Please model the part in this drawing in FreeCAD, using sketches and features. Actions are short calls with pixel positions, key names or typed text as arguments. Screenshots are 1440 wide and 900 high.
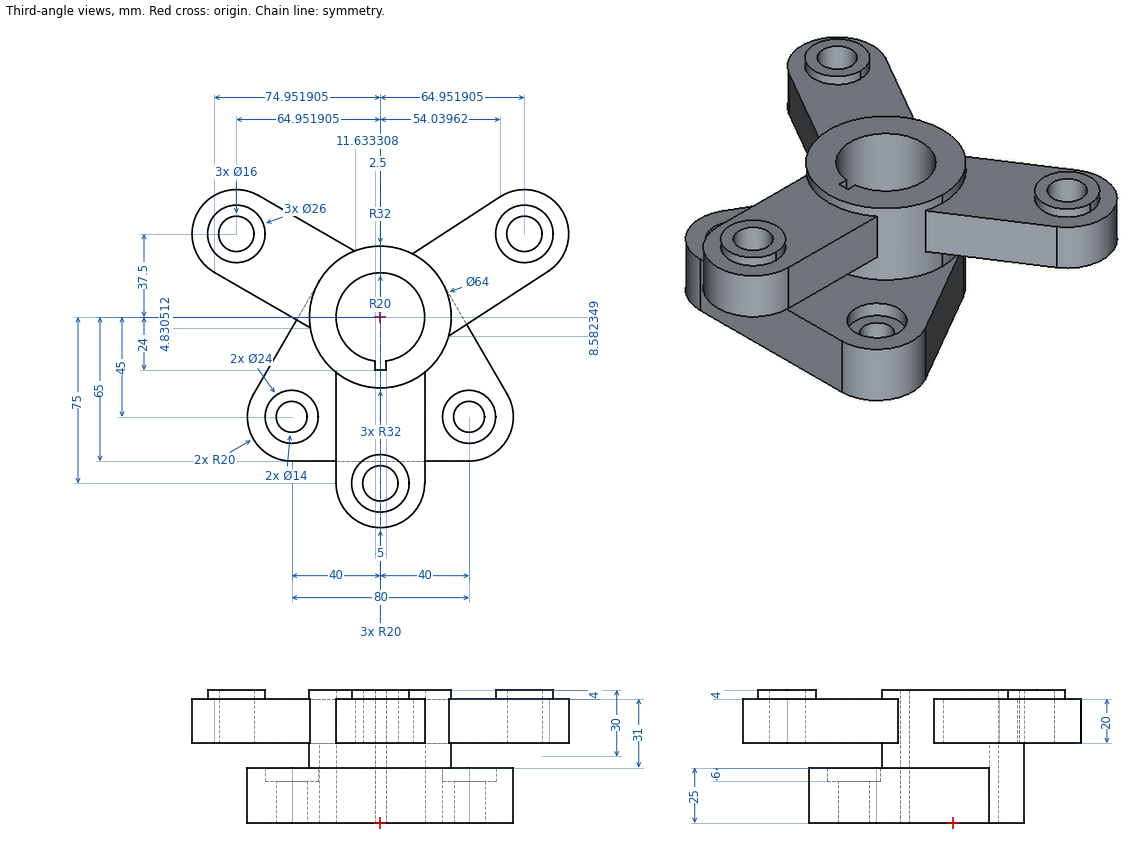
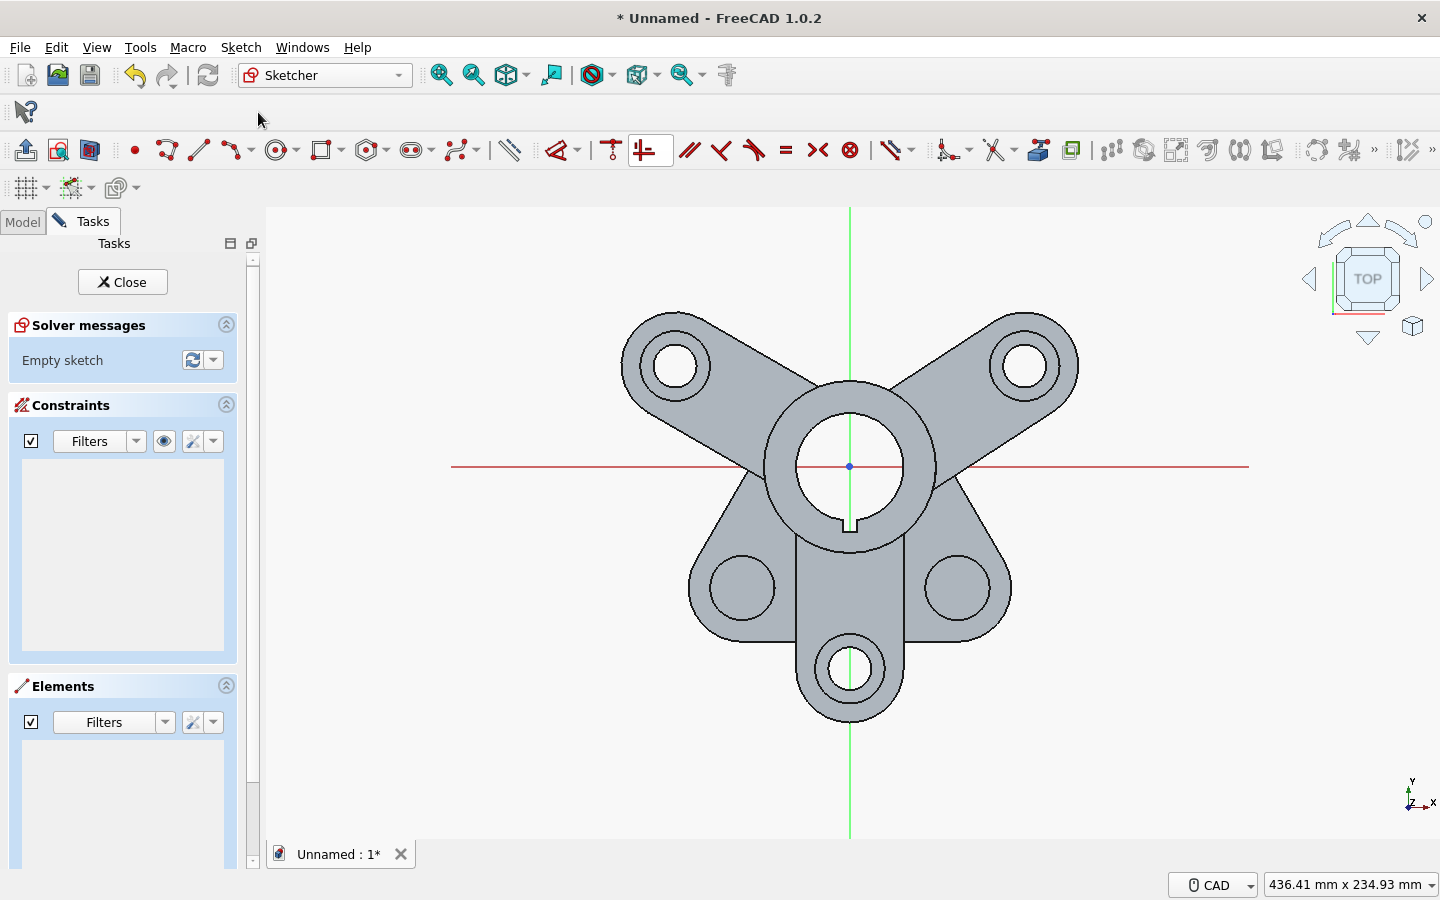
scroll(888, 545, up, 5)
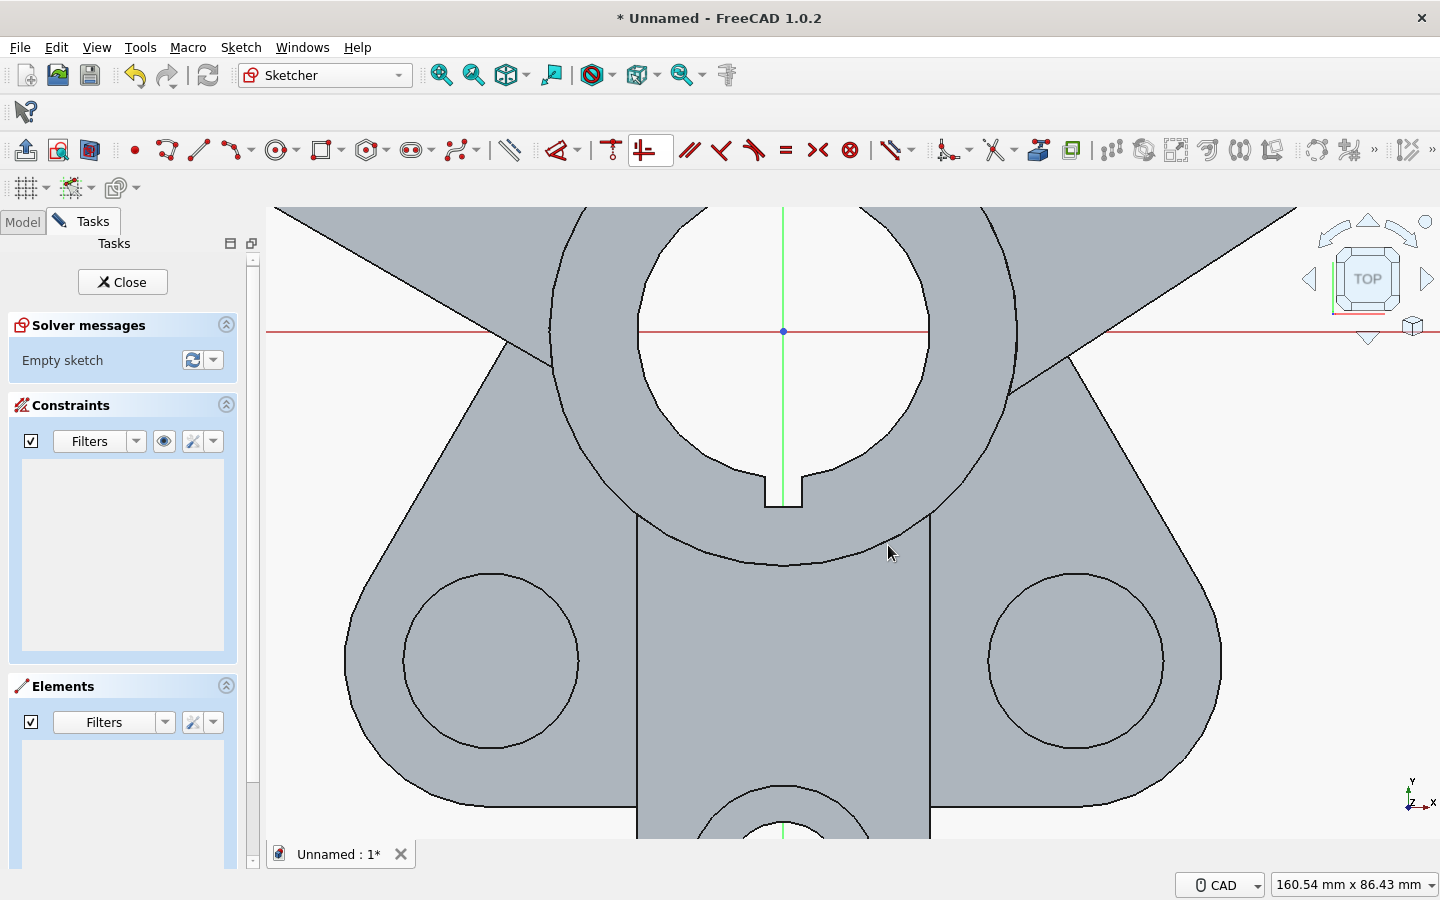
key(g)
key(c)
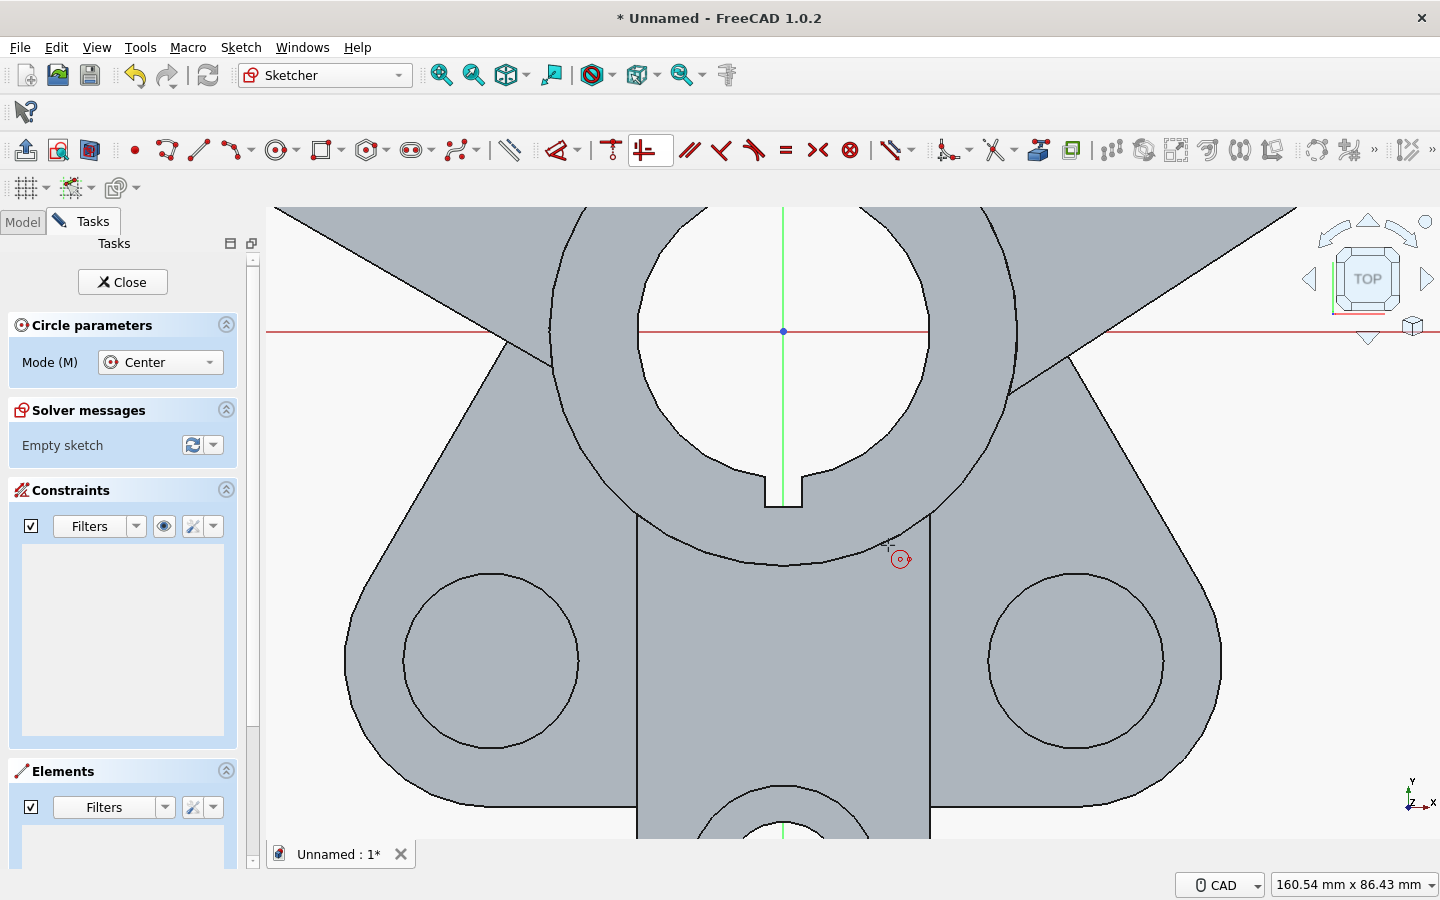
click(491, 661)
move(527, 625)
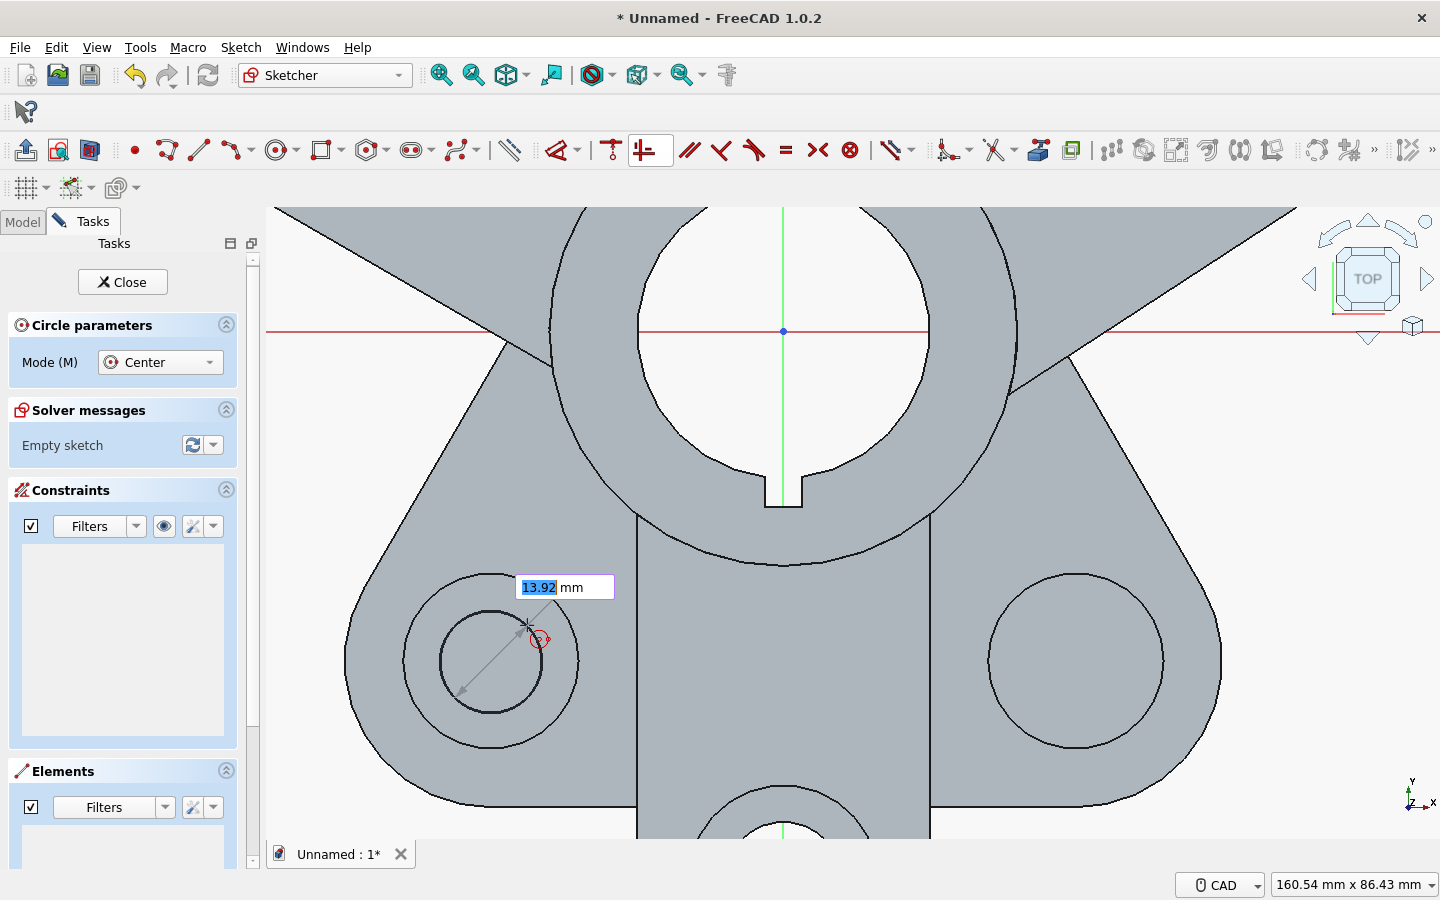
text(14)
key(Return)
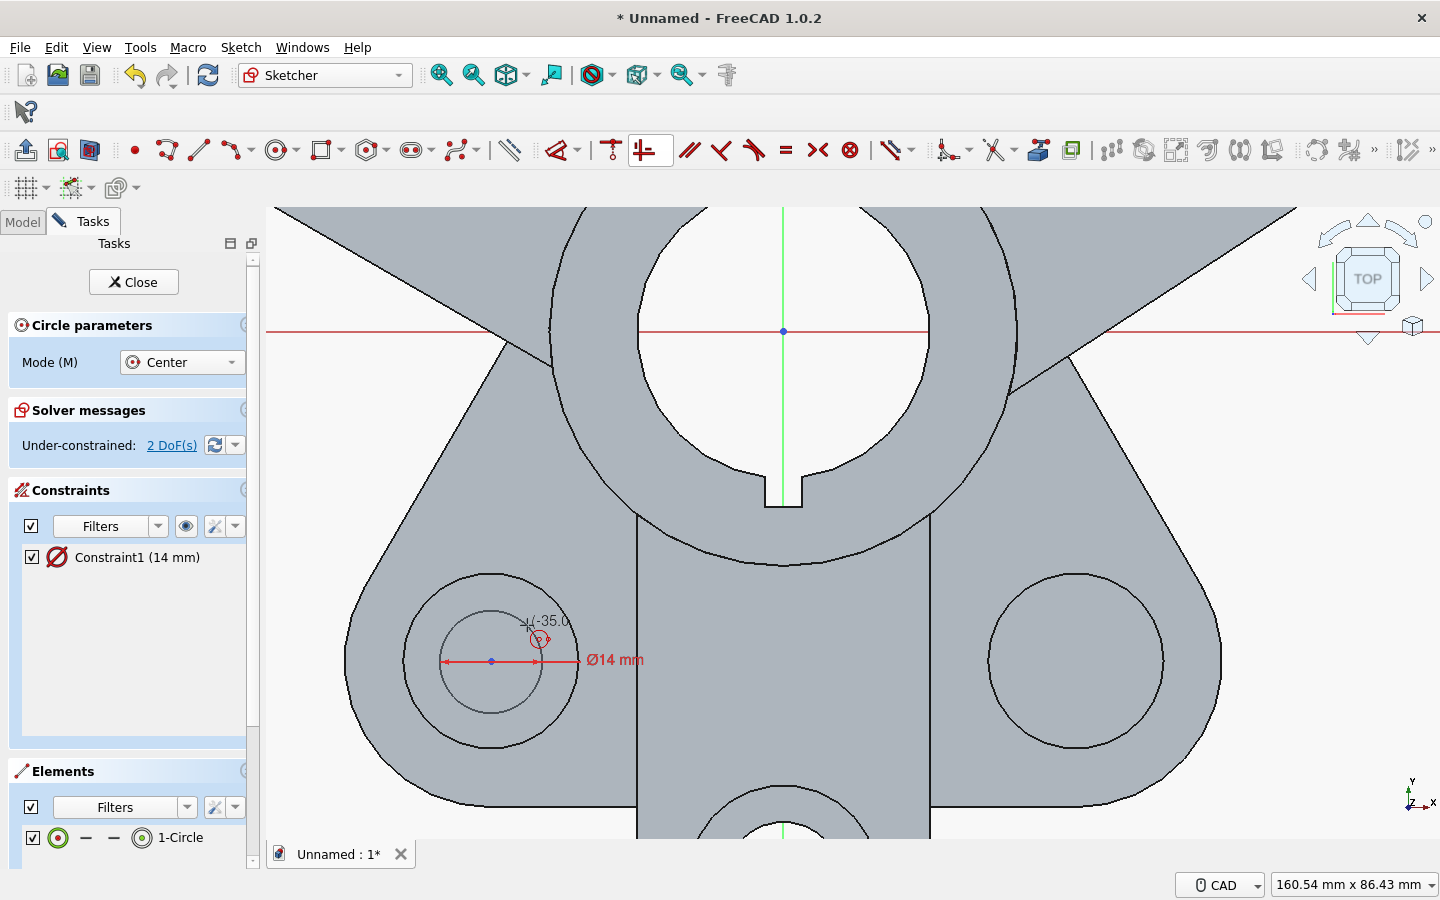
click(1076, 661)
move(1112, 625)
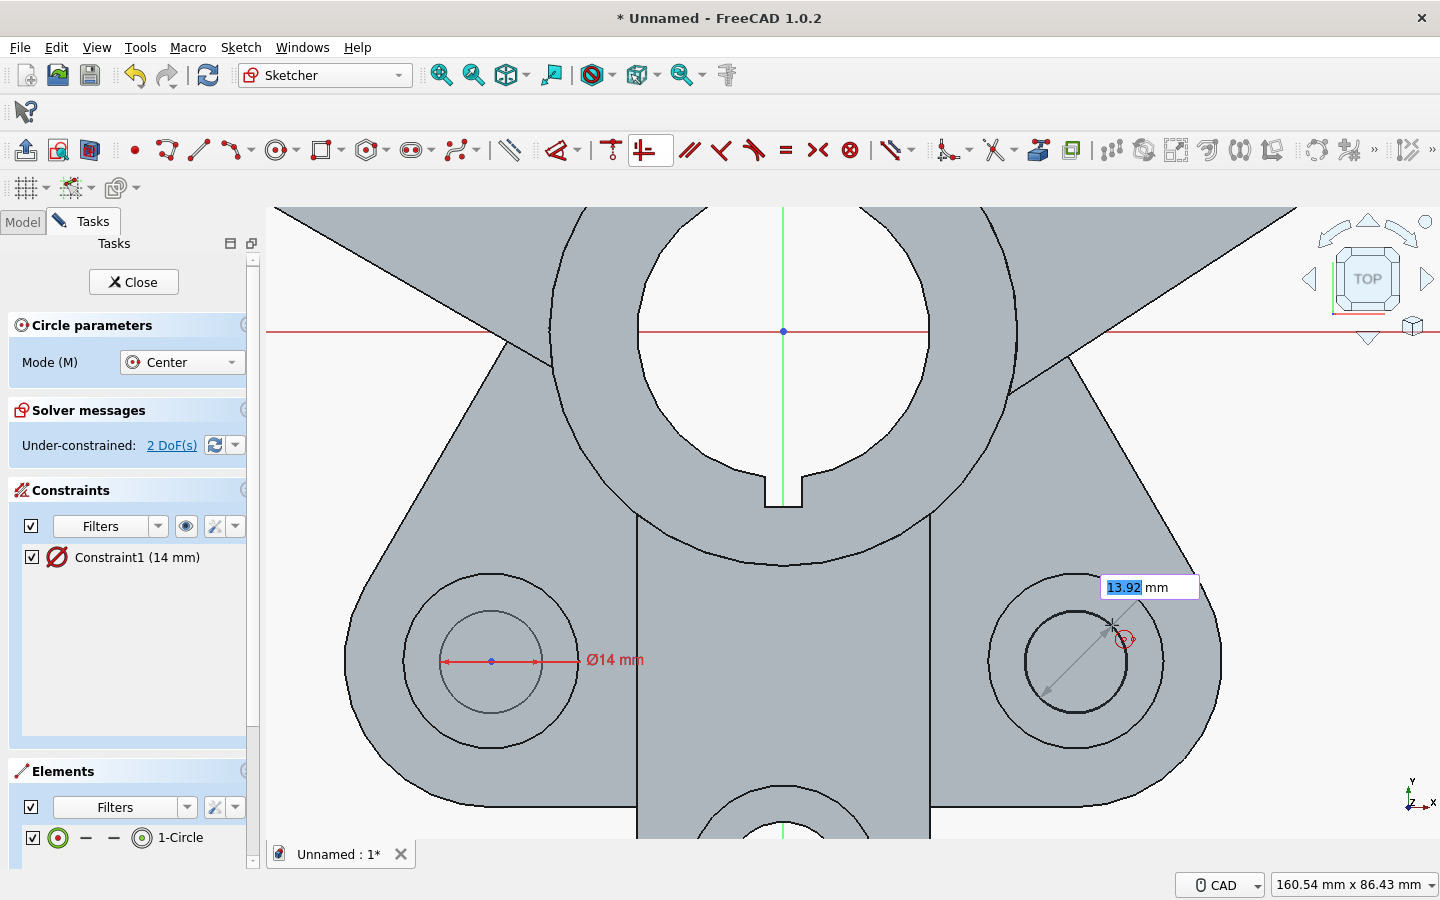
text(14)
key(Return)
key(Escape)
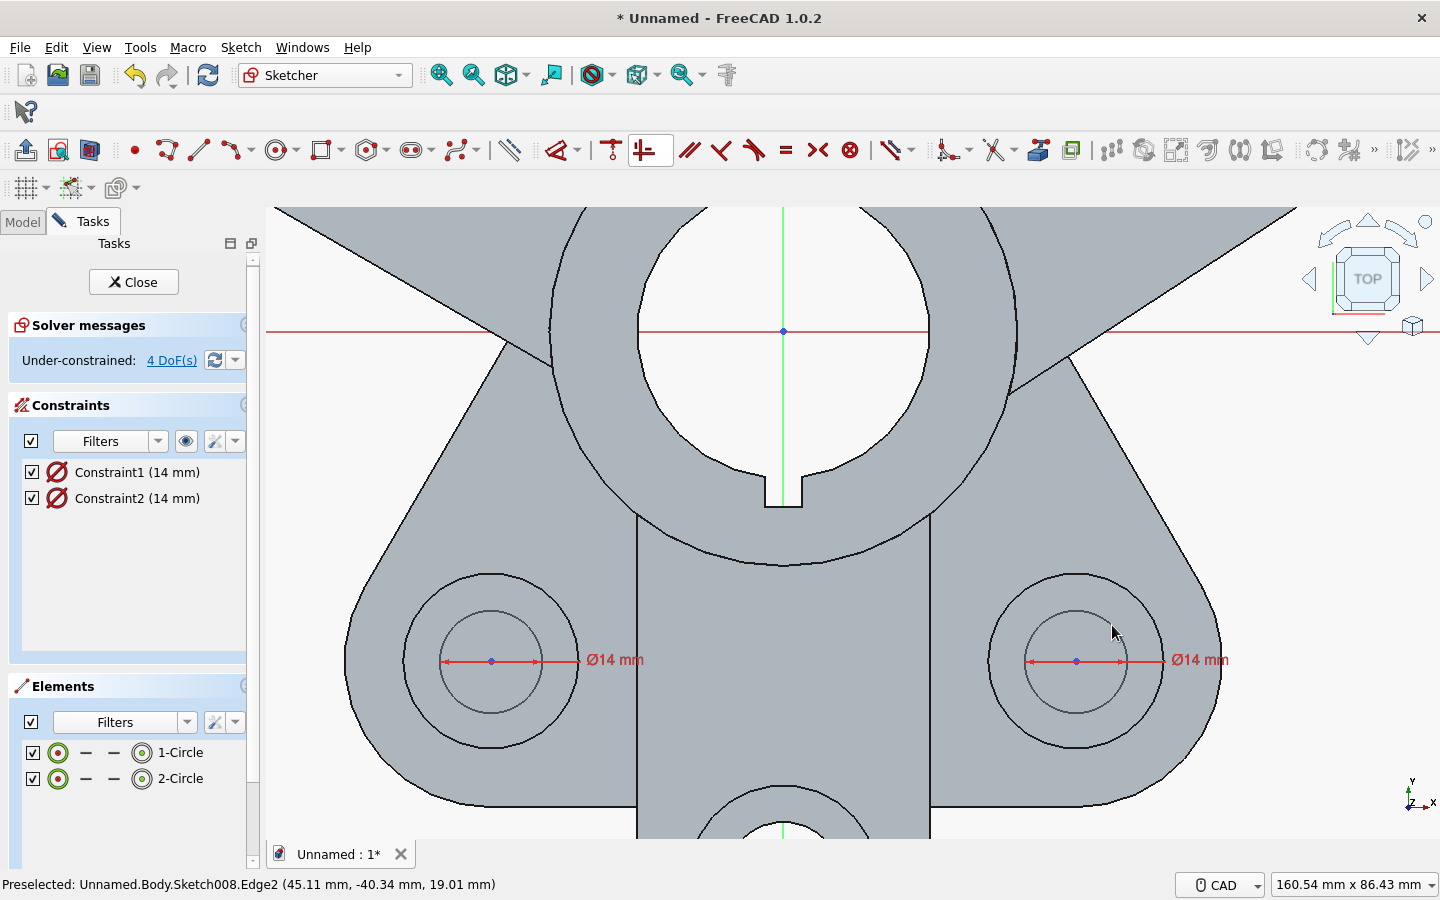
click(491, 662)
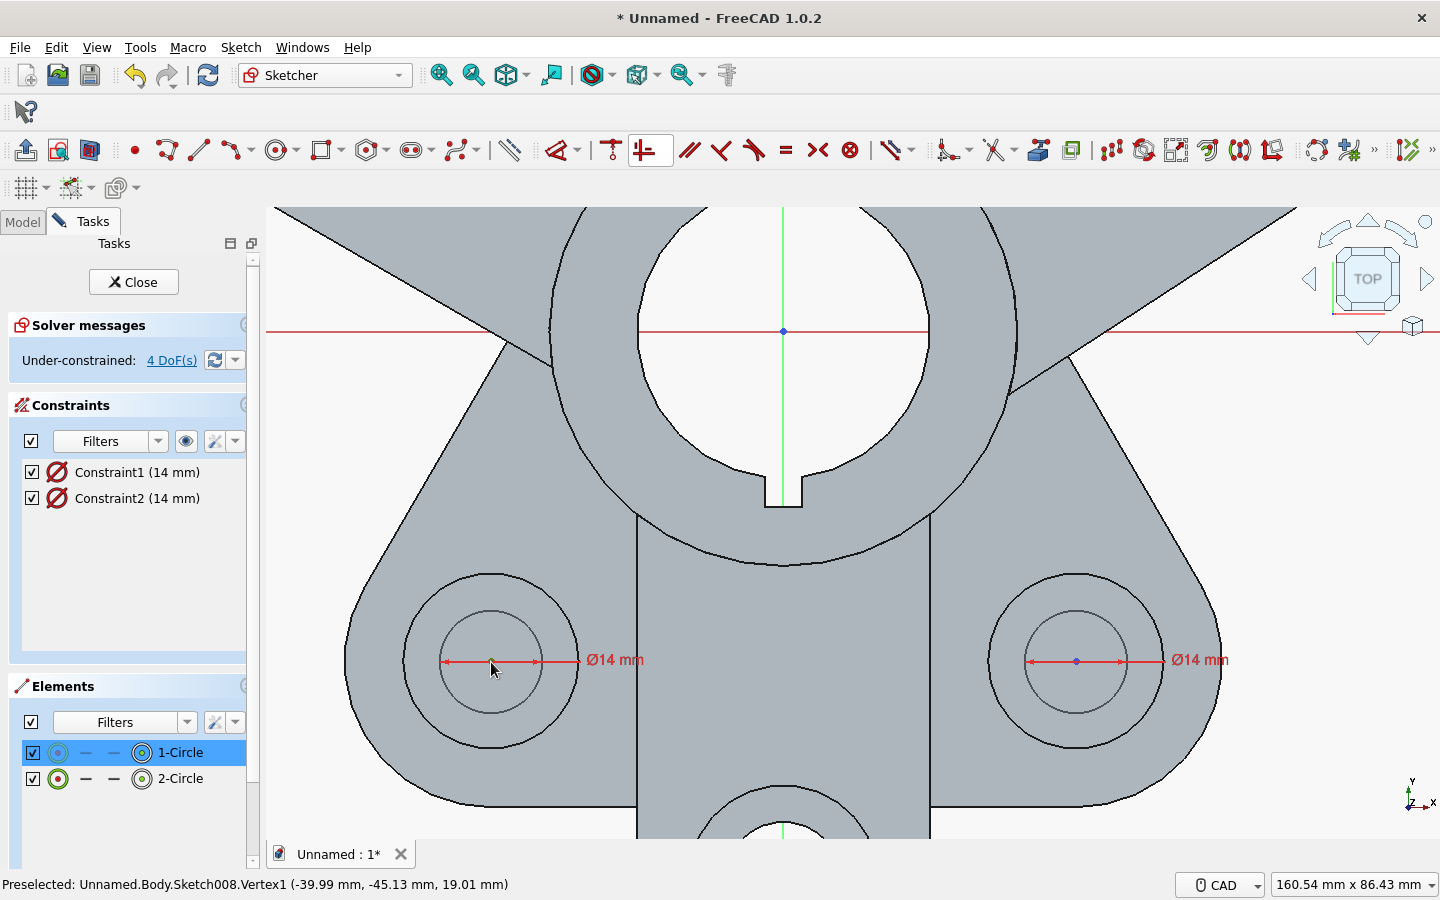
click(1076, 662)